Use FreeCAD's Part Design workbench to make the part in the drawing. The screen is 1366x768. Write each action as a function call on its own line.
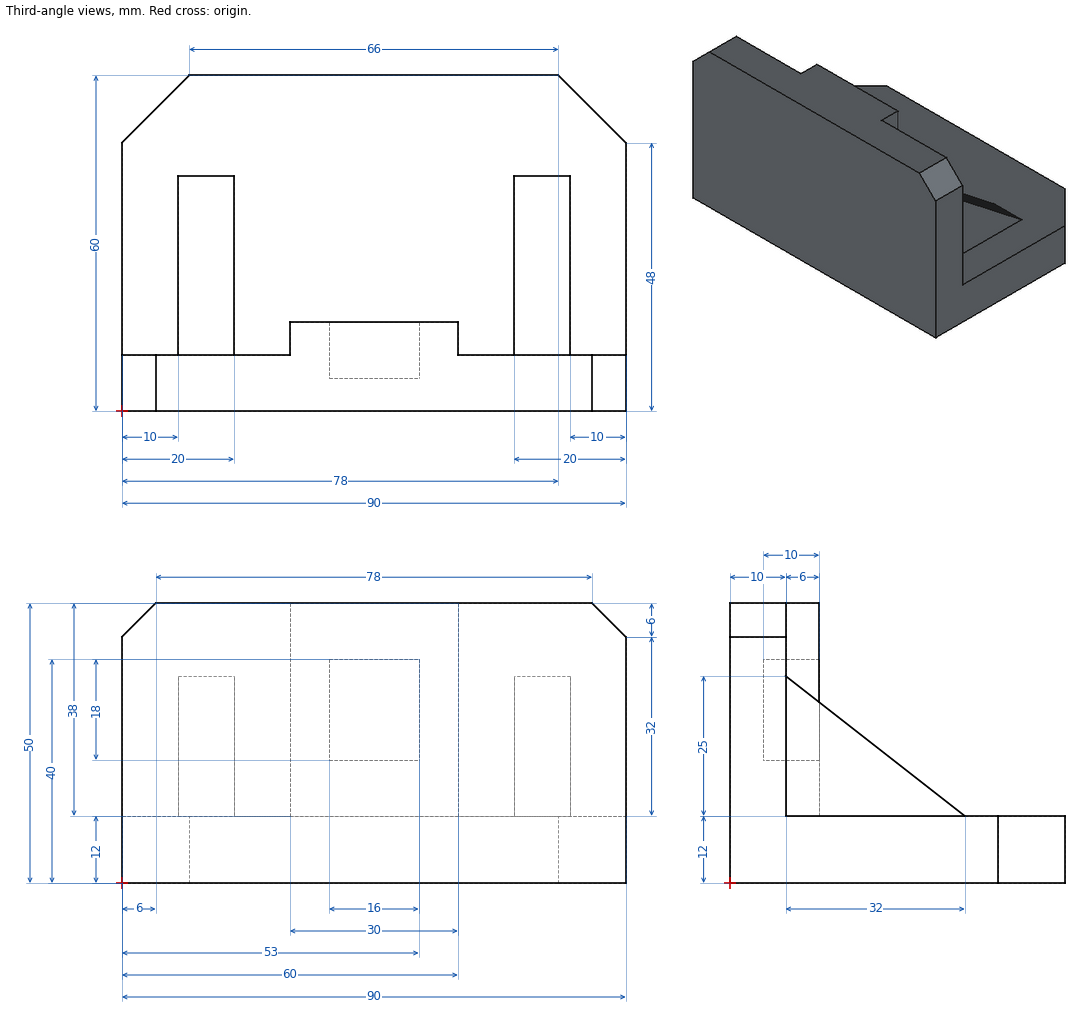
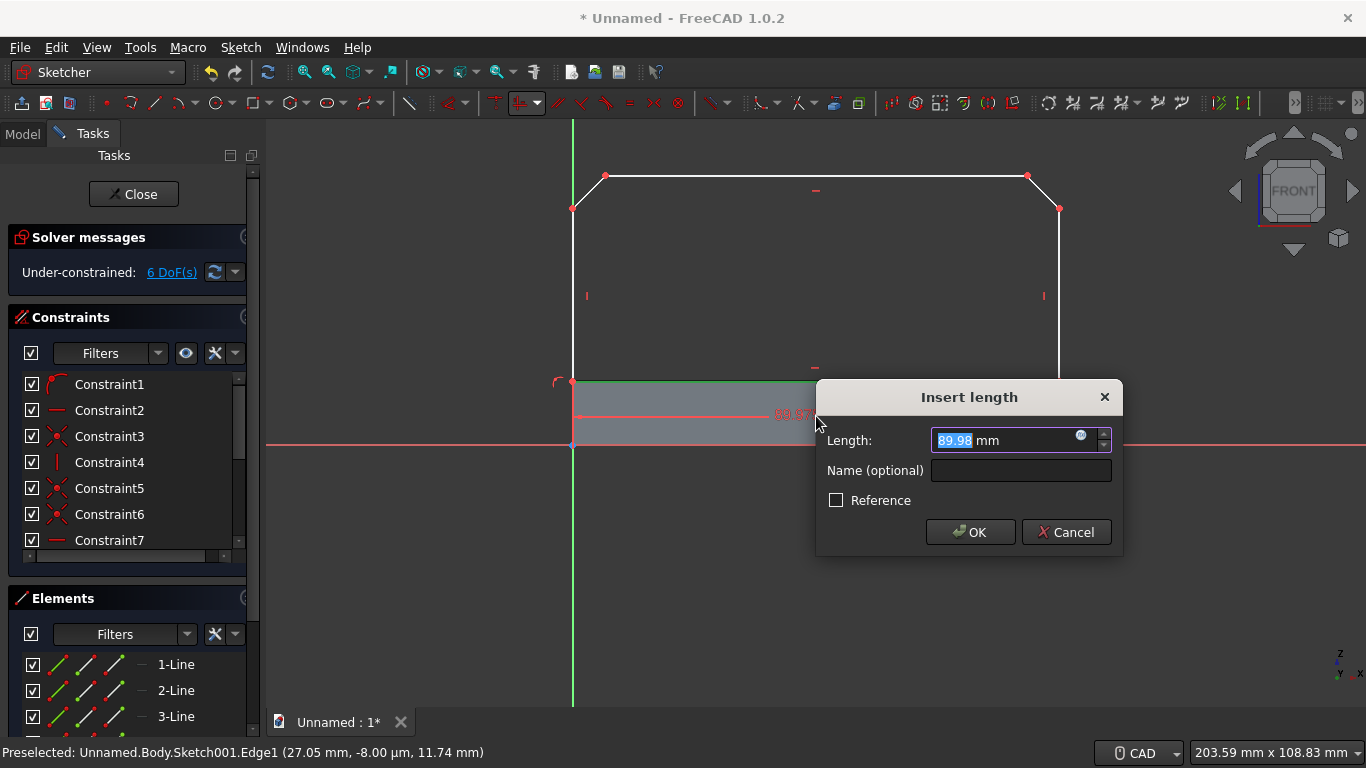
text(90)
key(Return)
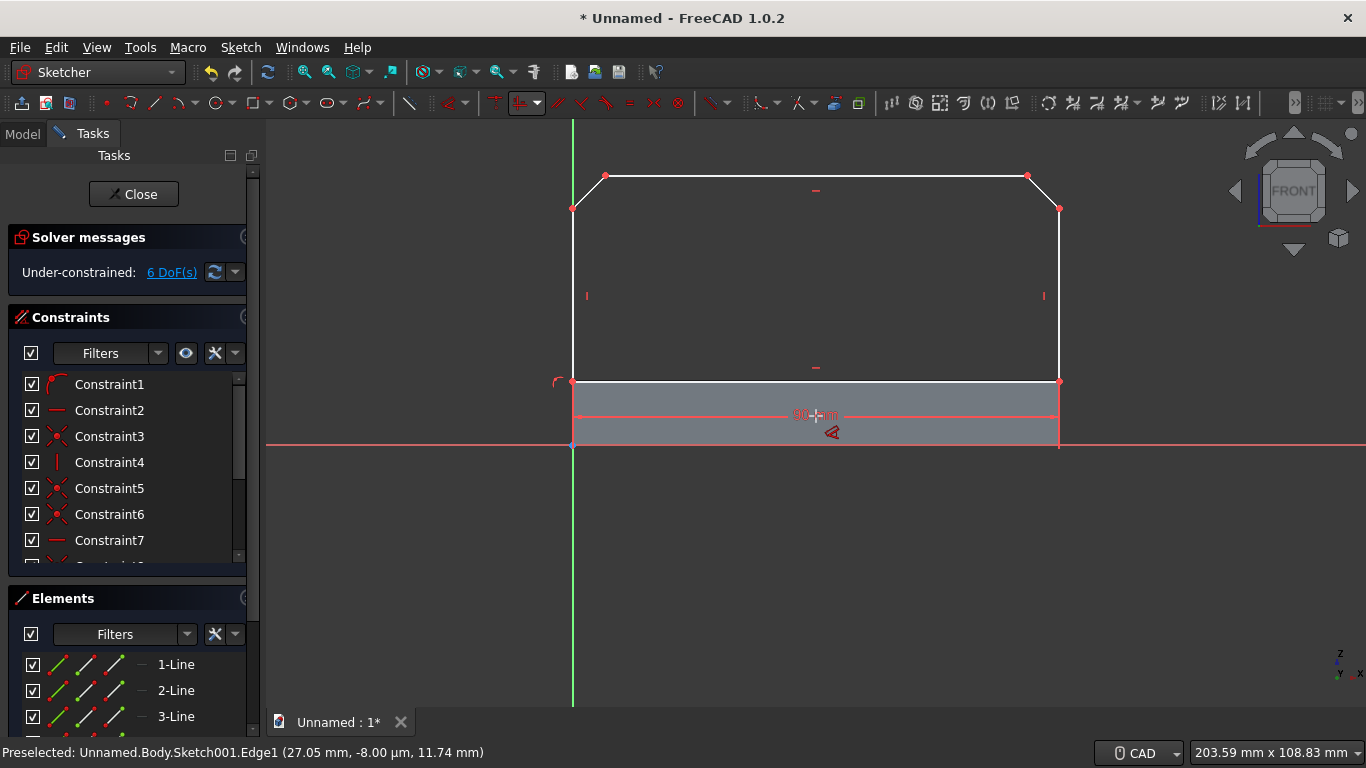
click(1059, 330)
click(1093, 295)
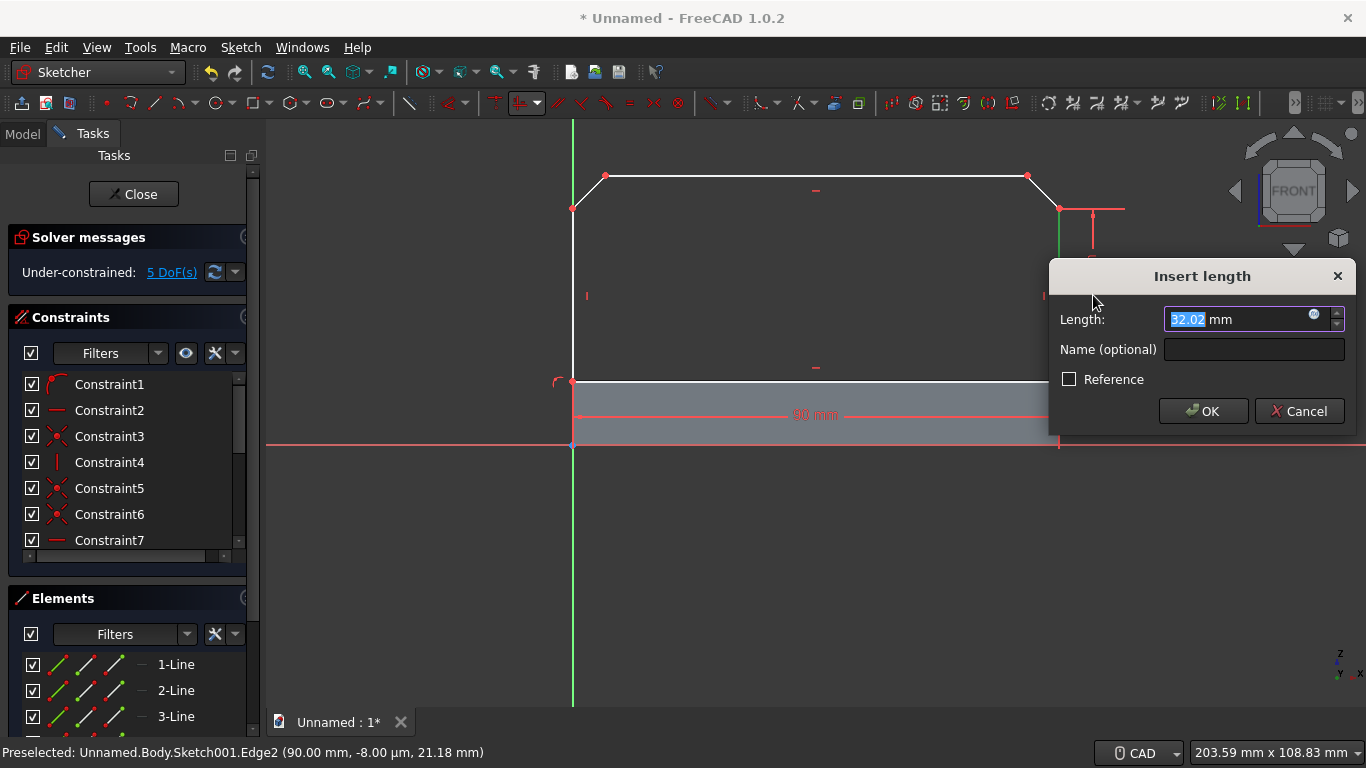
text(32)
key(Return)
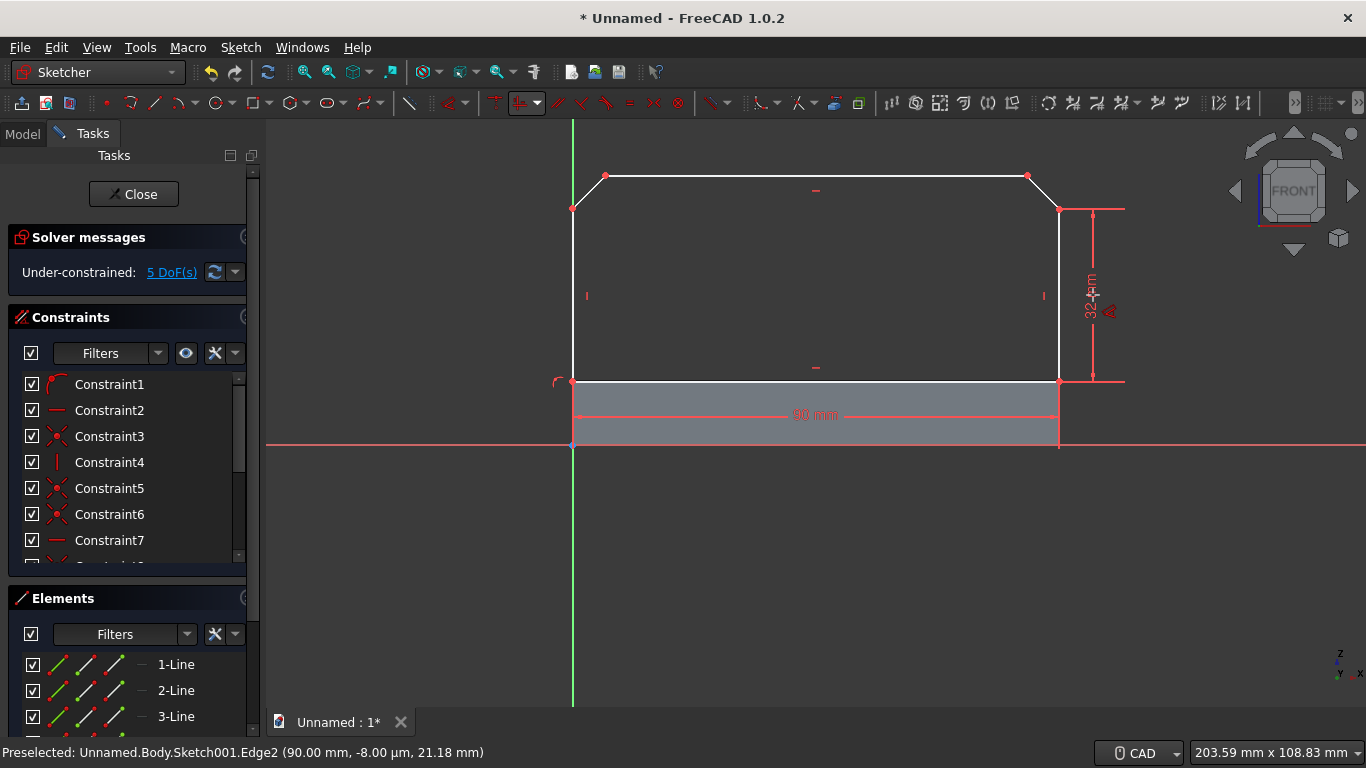
click(900, 176)
click(816, 210)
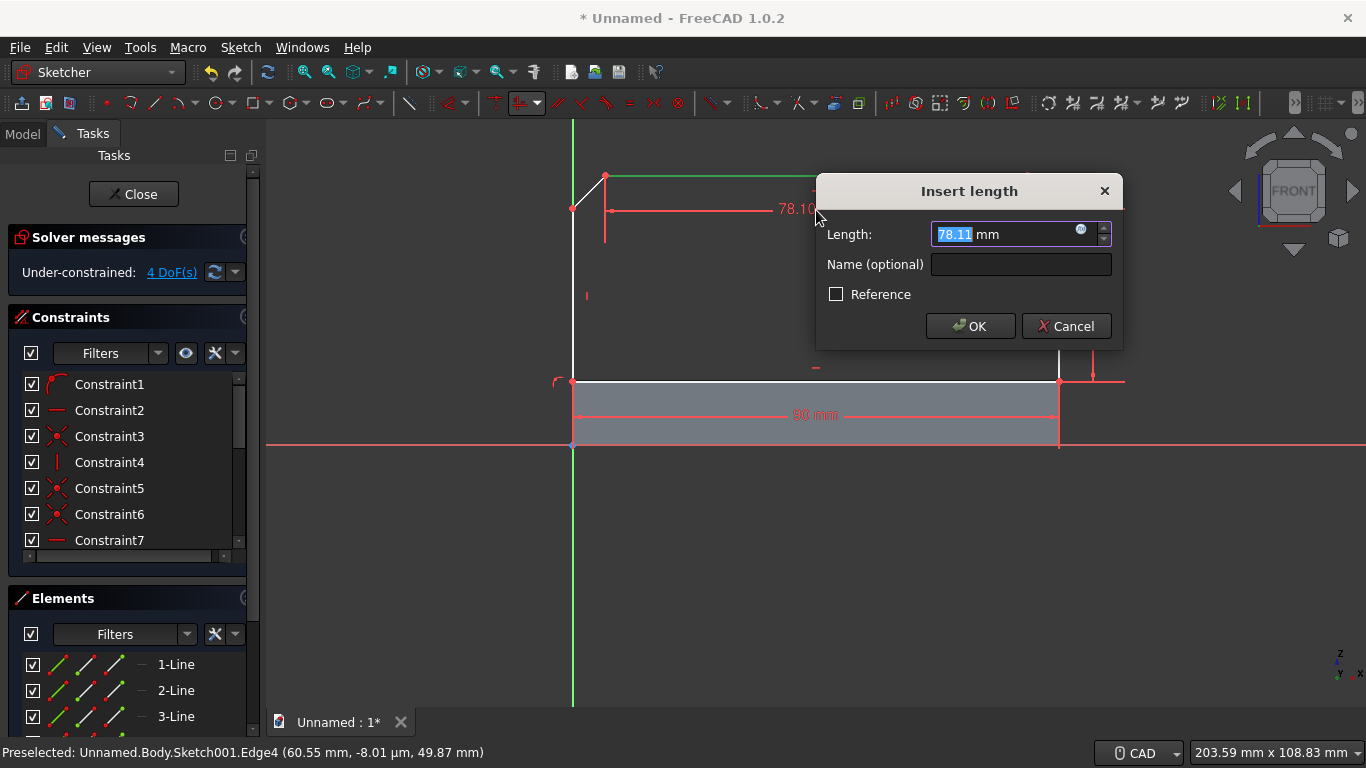
text(78)
key(Return)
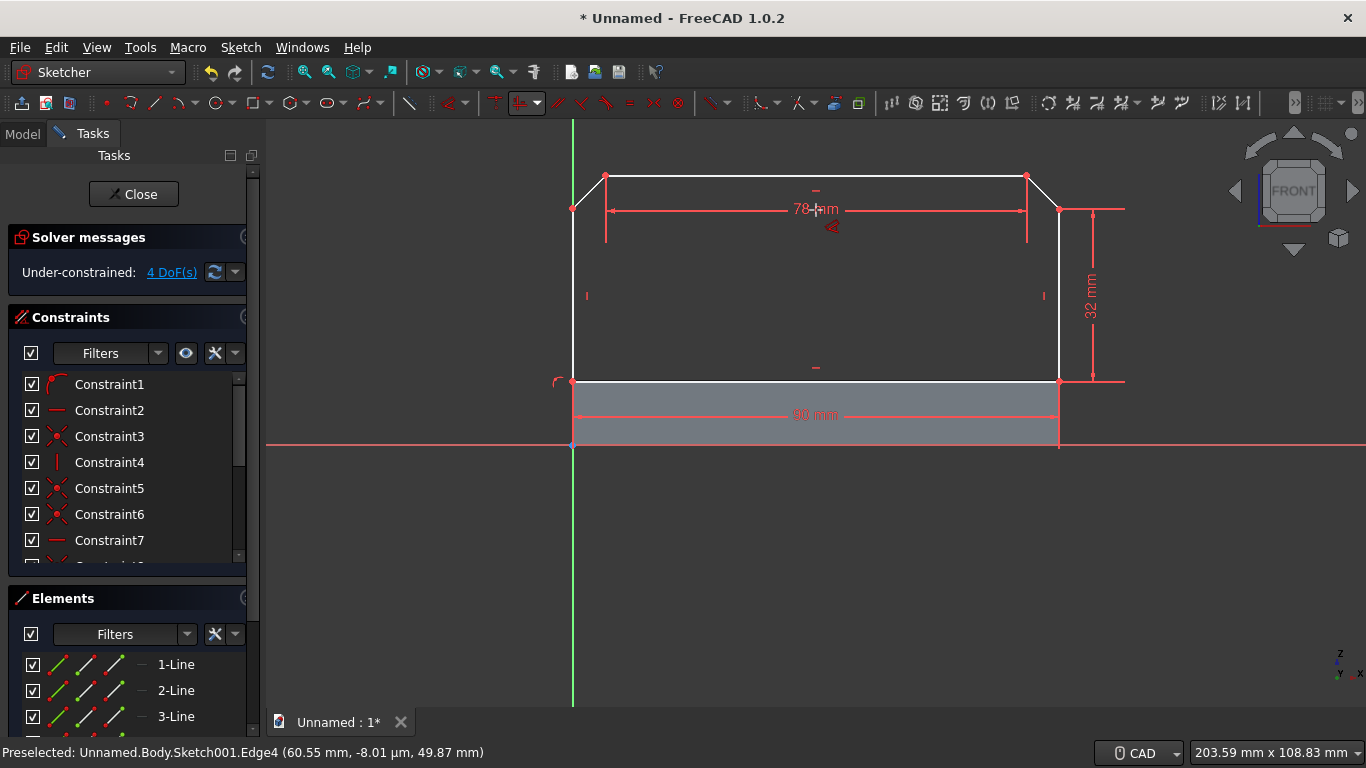
click(573, 261)
click(539, 295)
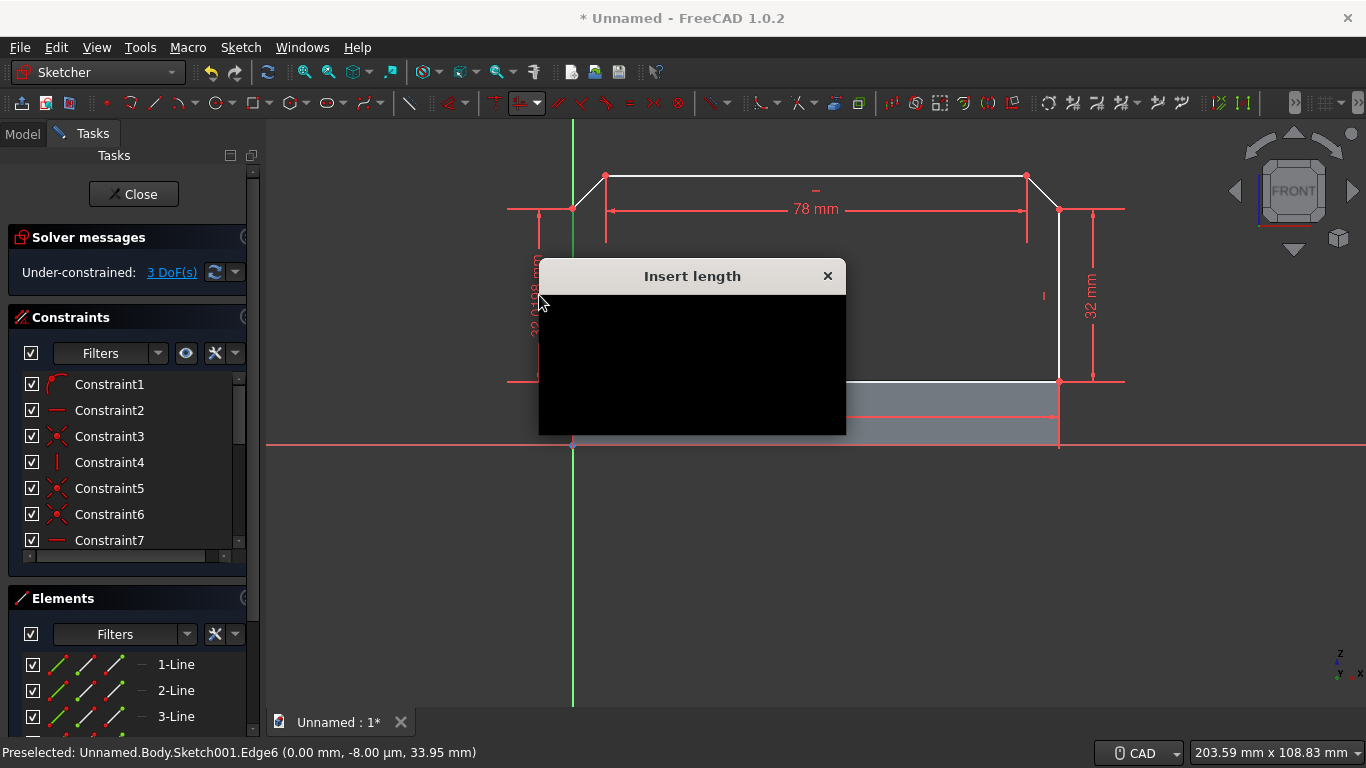
text(32)
key(Return)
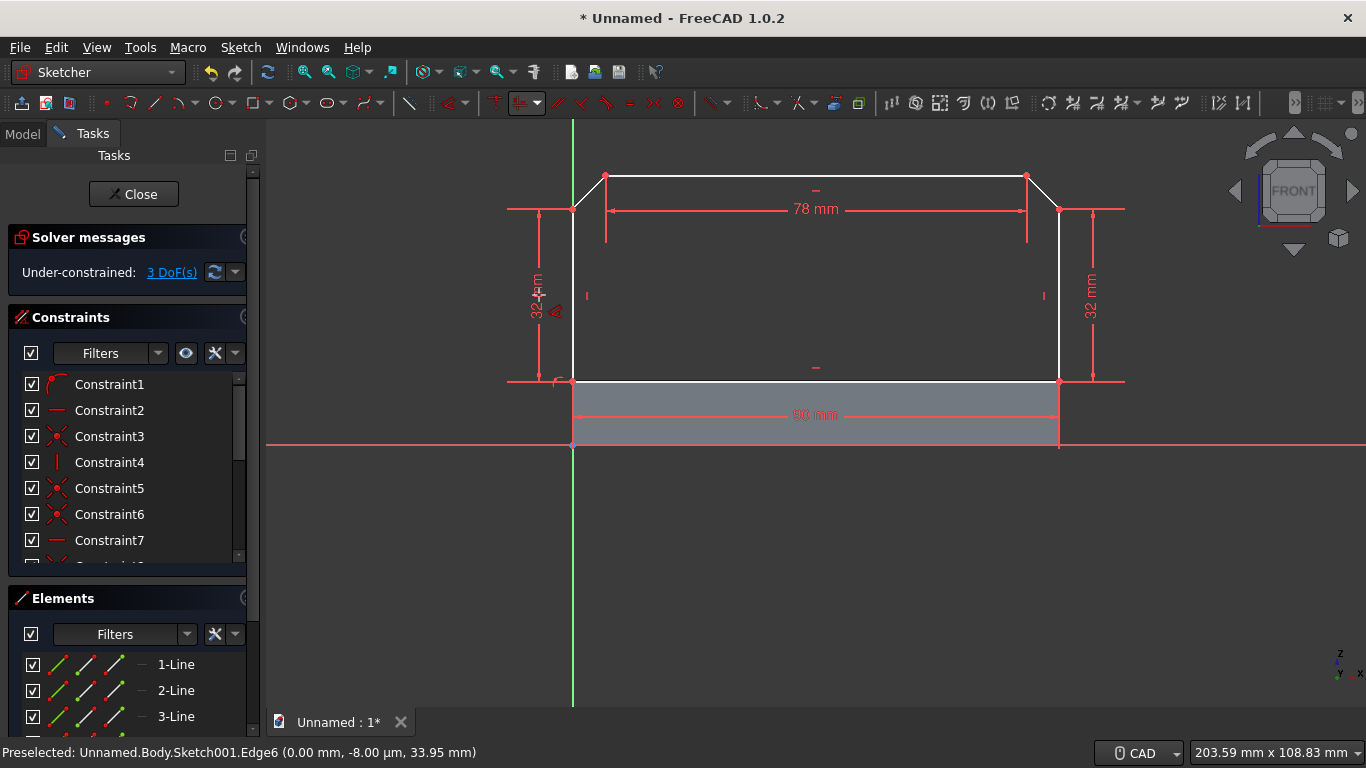
scroll(606, 176, up, 2)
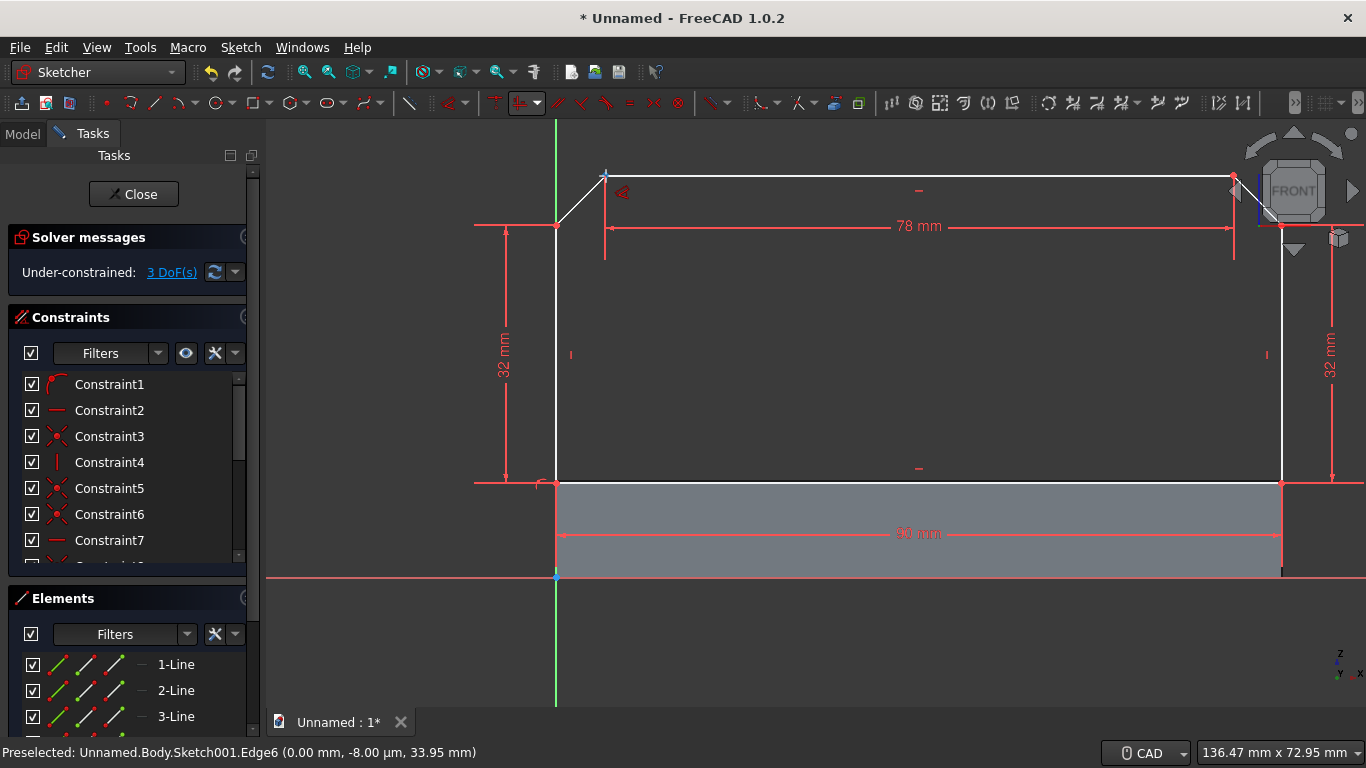
click(605, 176)
click(581, 612)